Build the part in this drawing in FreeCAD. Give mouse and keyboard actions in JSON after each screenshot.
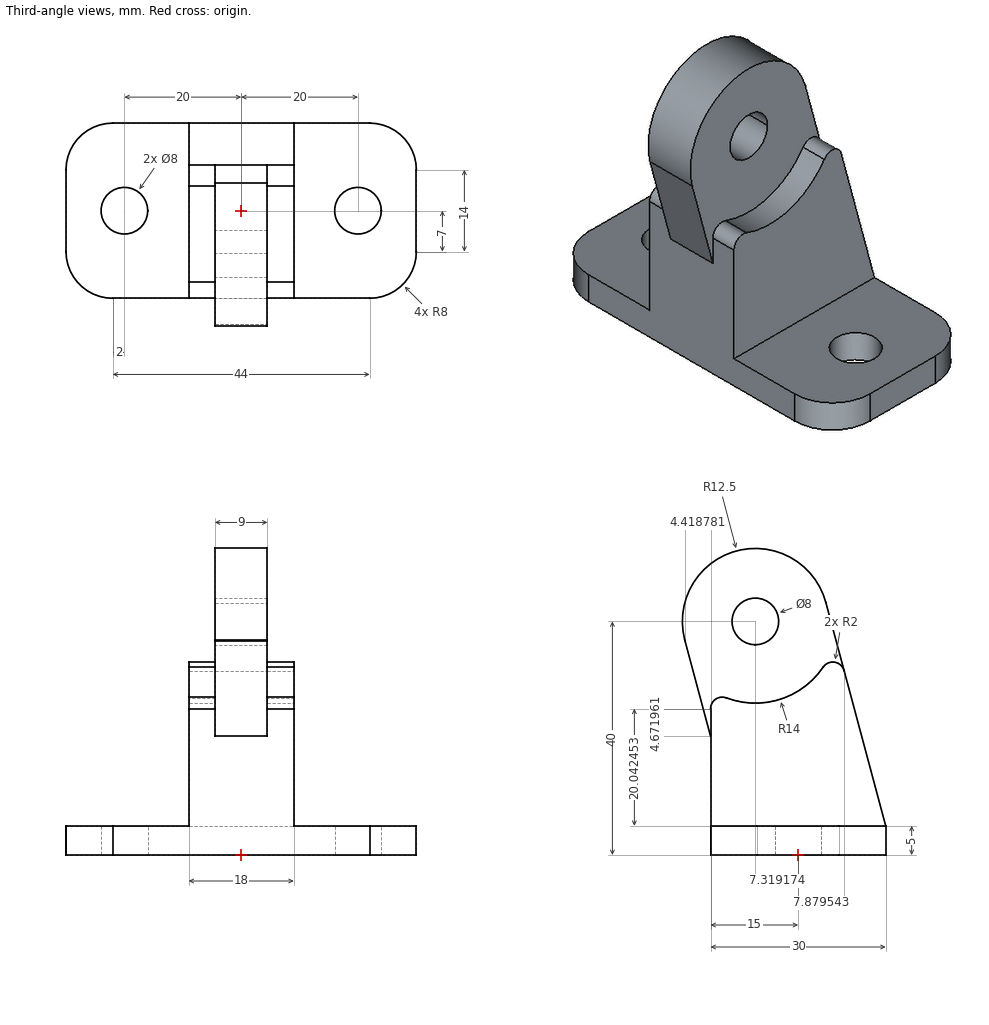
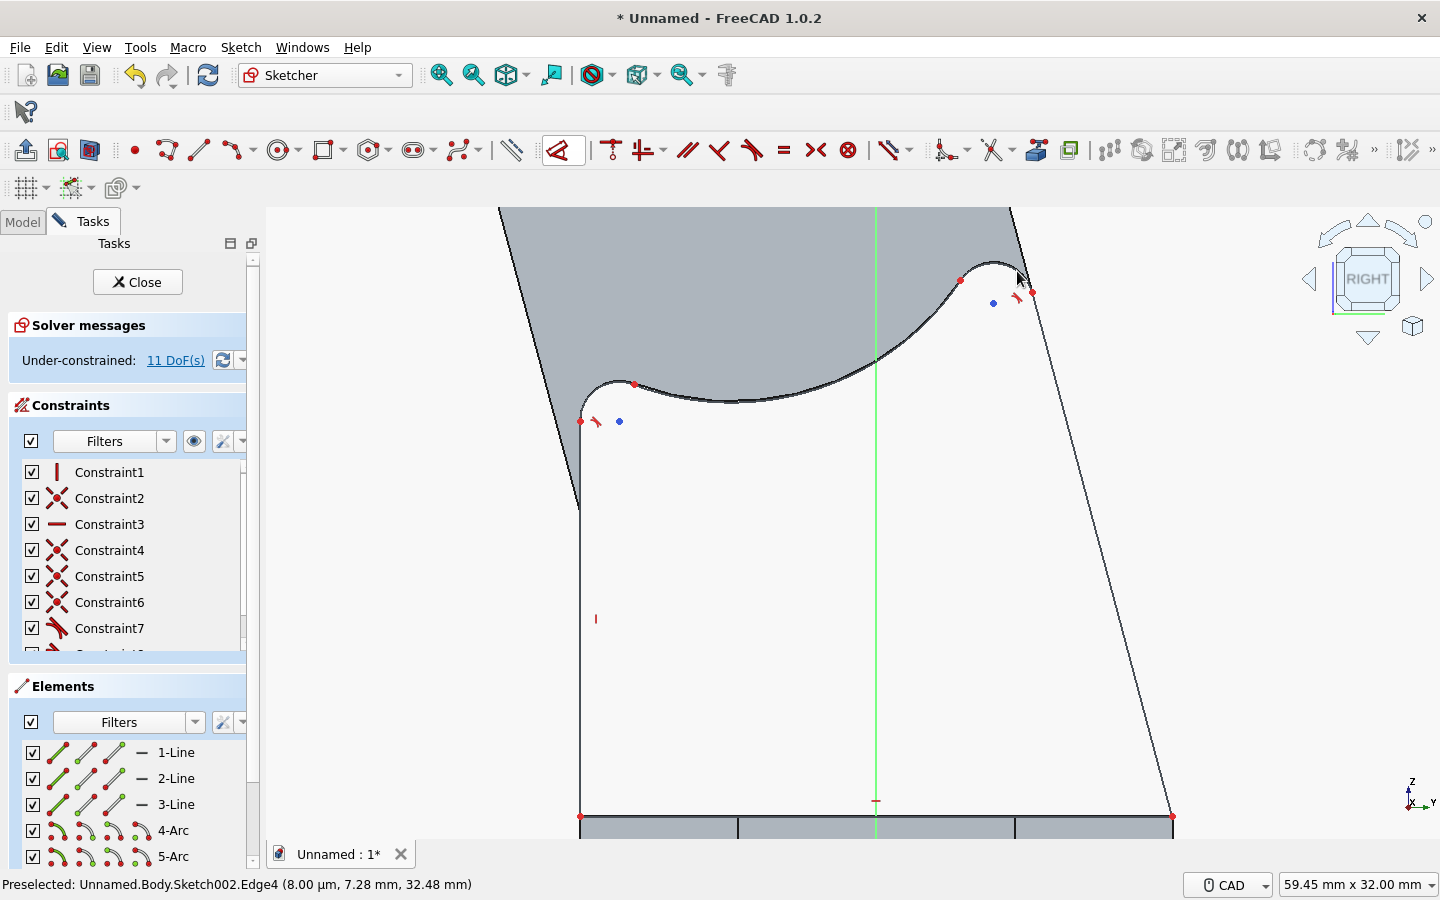
{"action": "left_click", "coordinate": [1017, 271]}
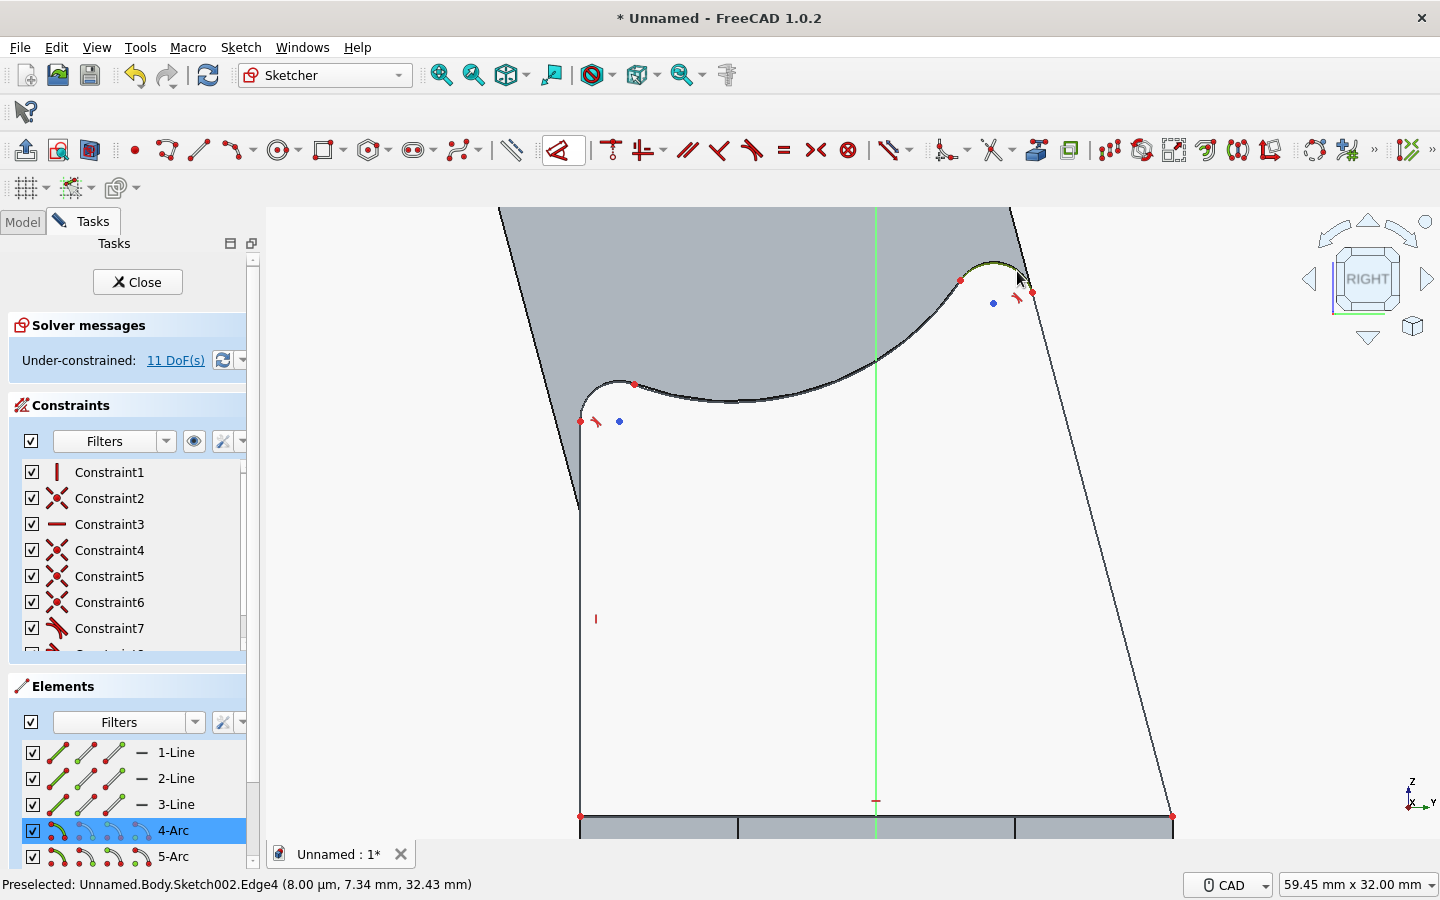
{"action": "left_click", "coordinate": [743, 402]}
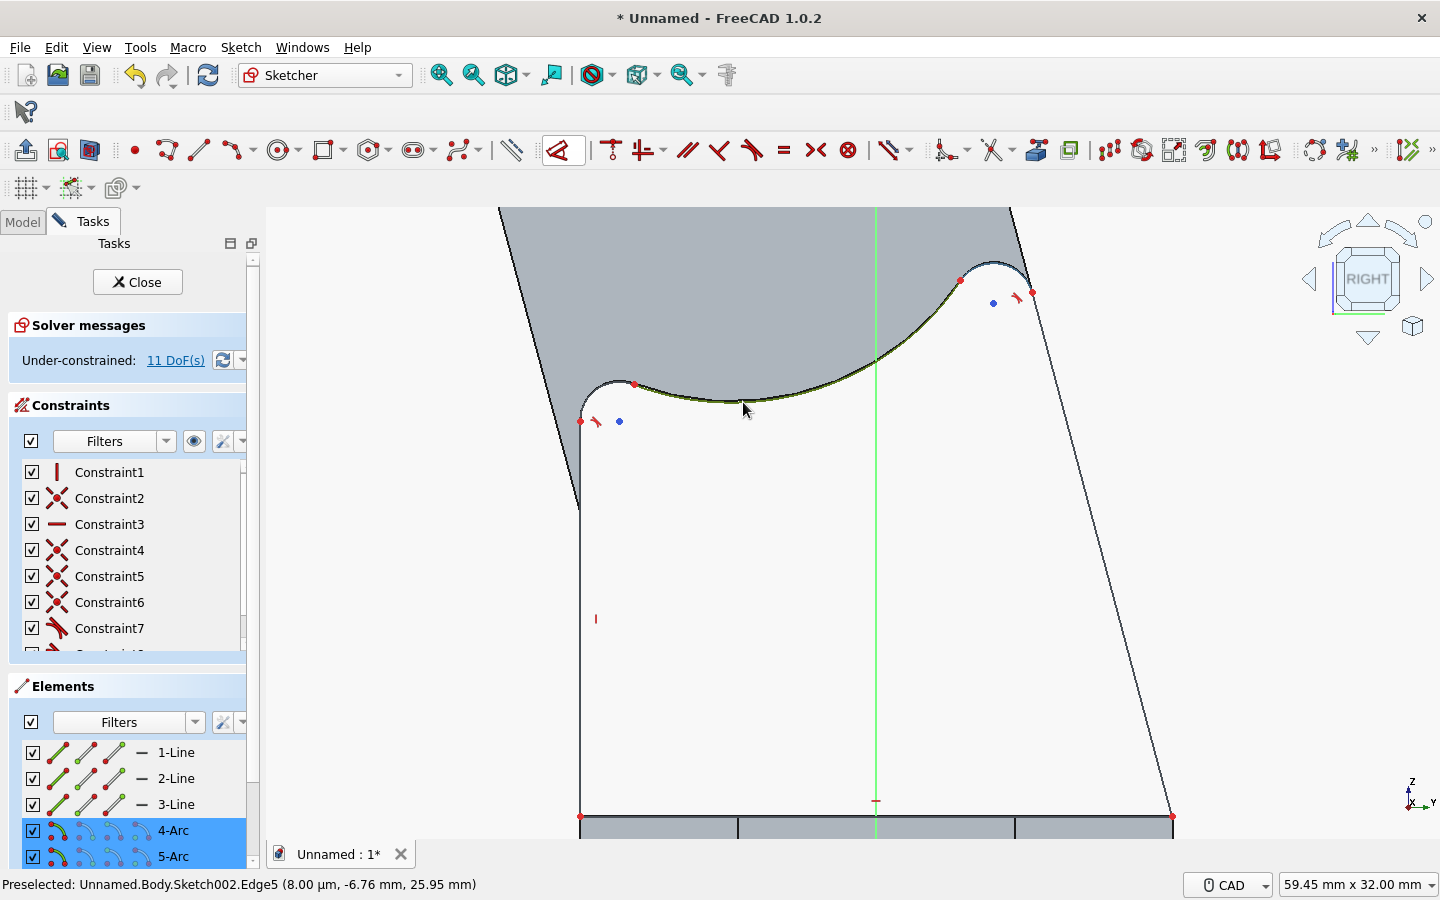
{"action": "key", "text": "t"}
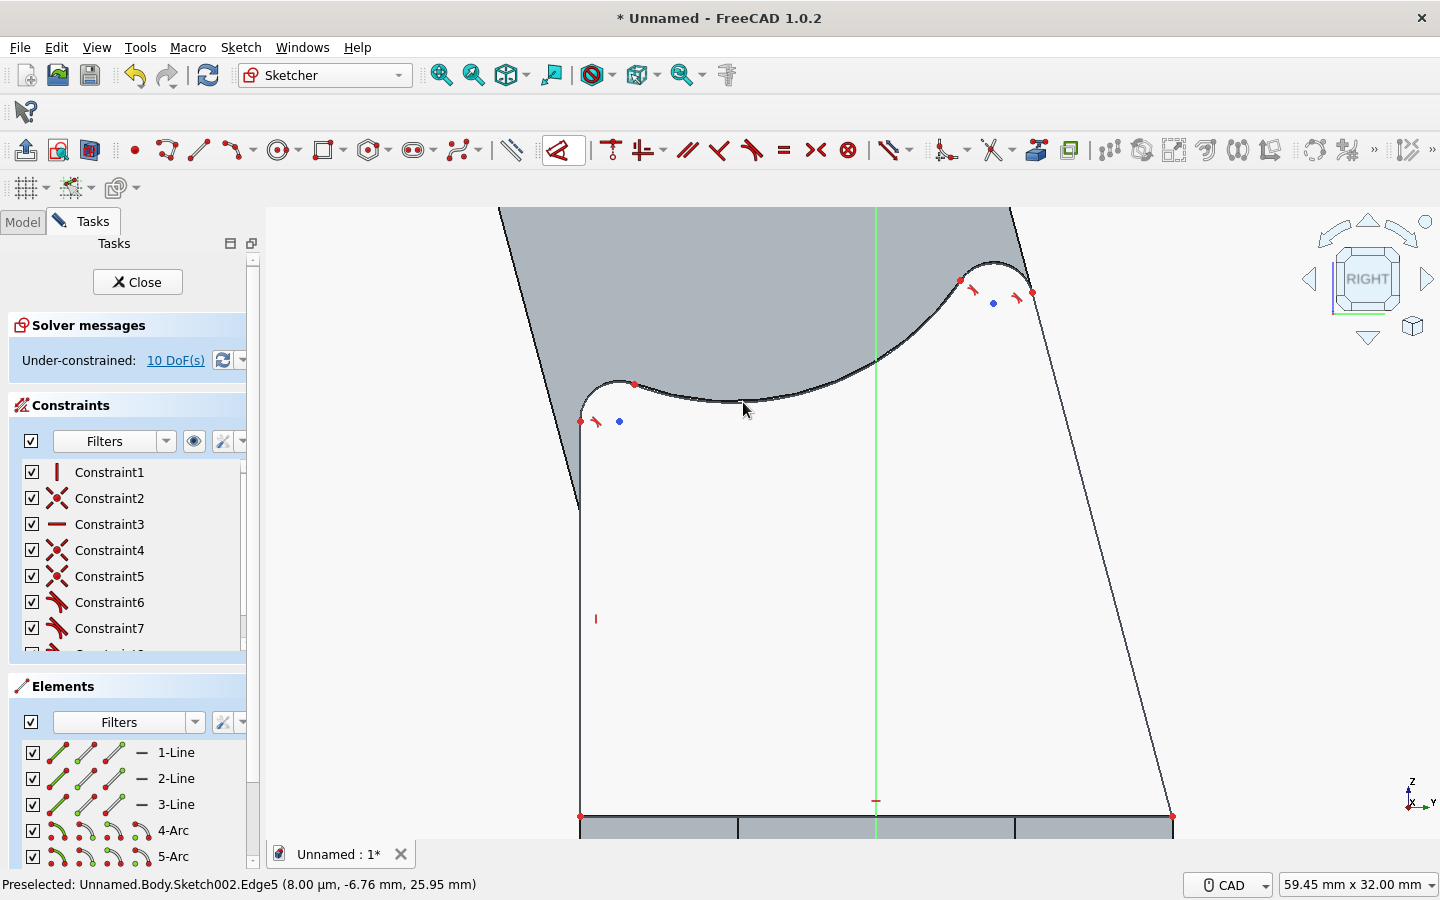
{"action": "left_click", "coordinate": [743, 402]}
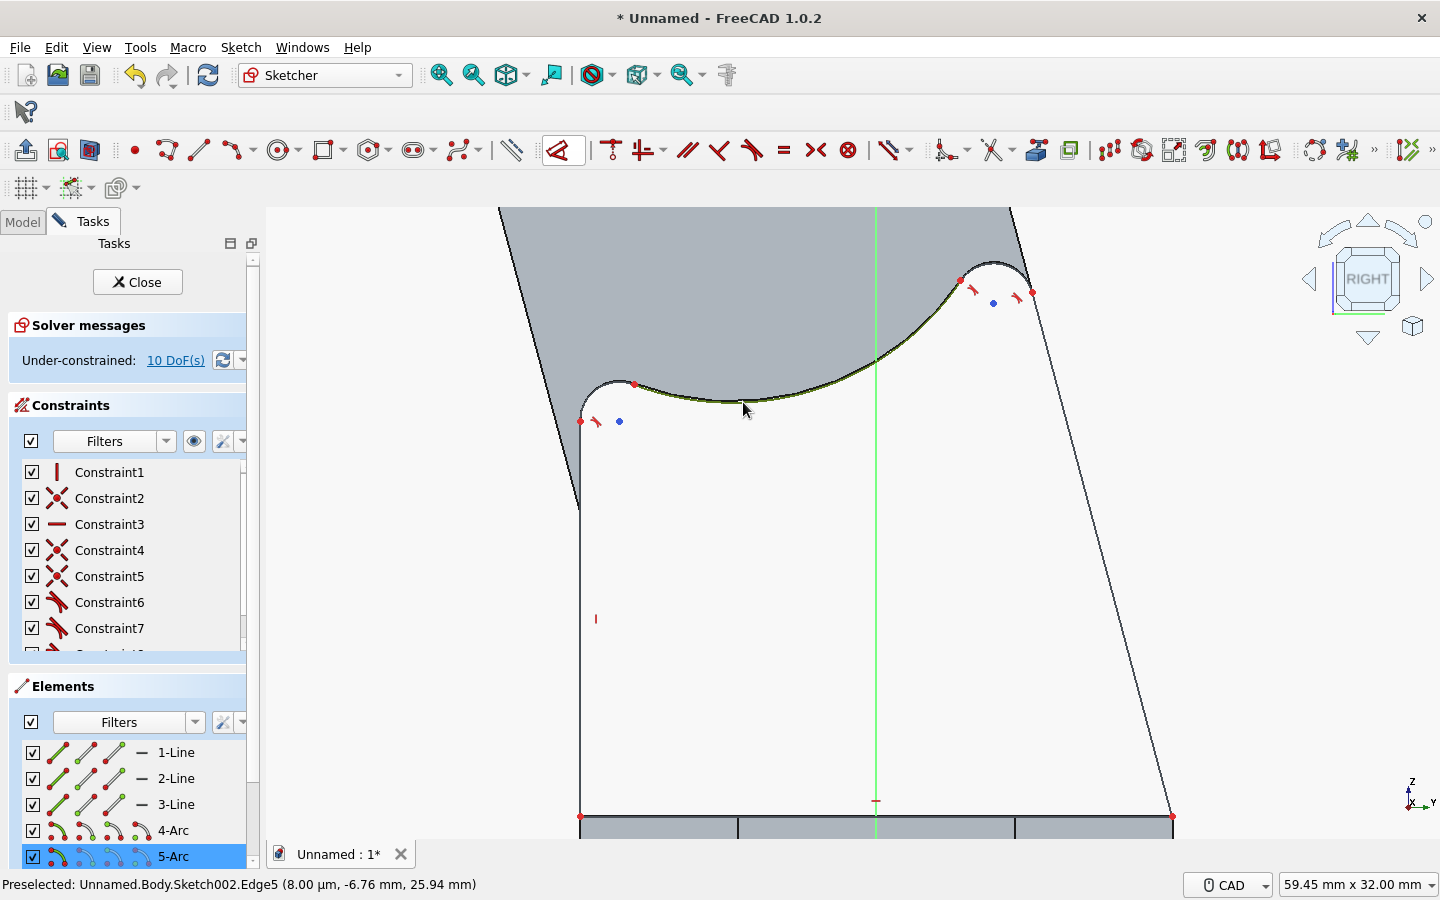
{"action": "left_click", "coordinate": [612, 383]}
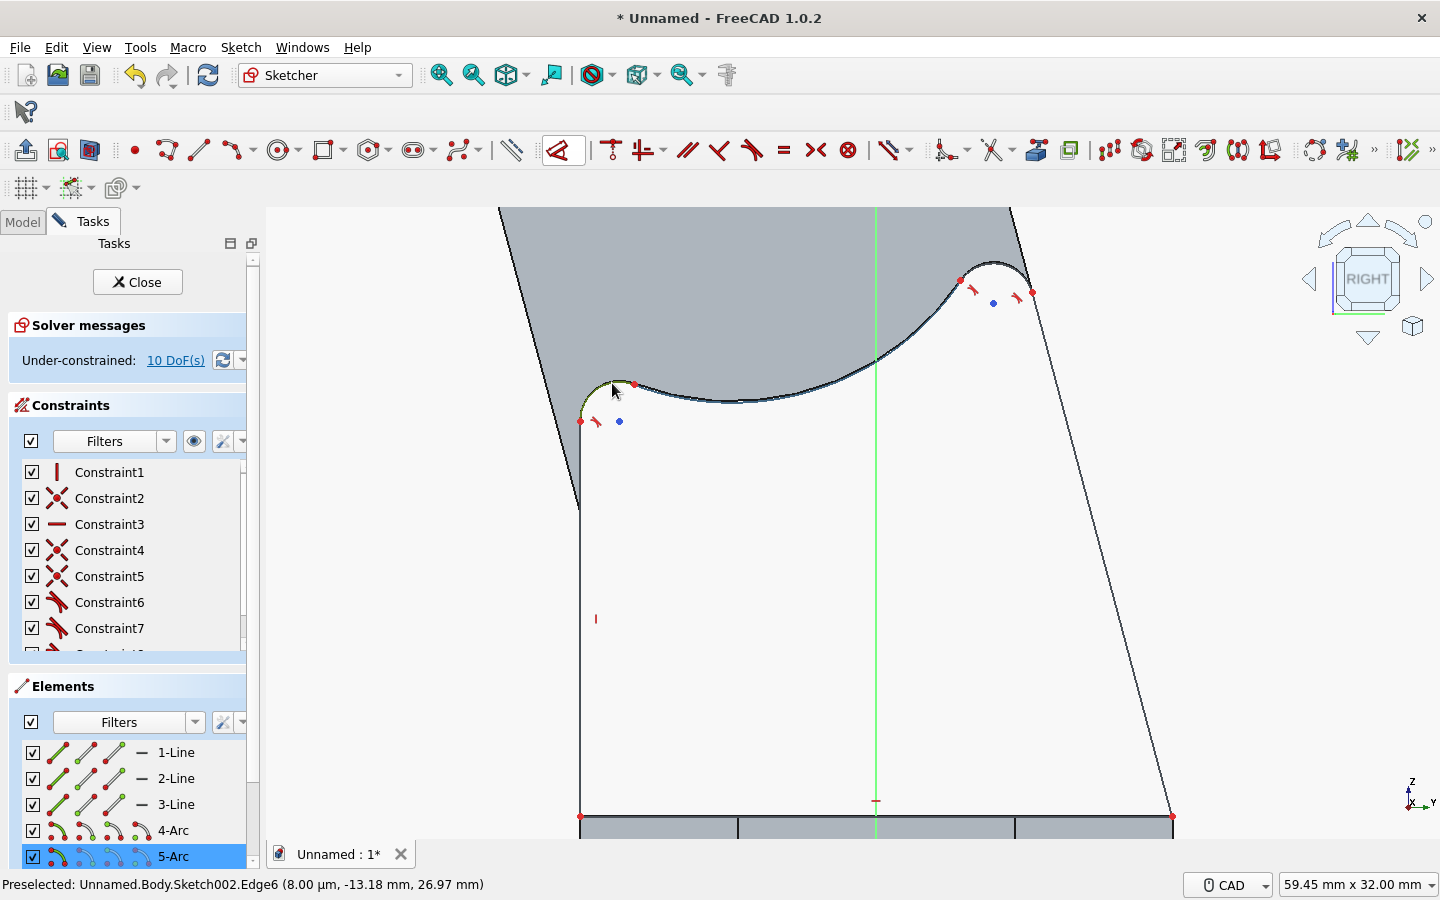
{"action": "key", "text": "t"}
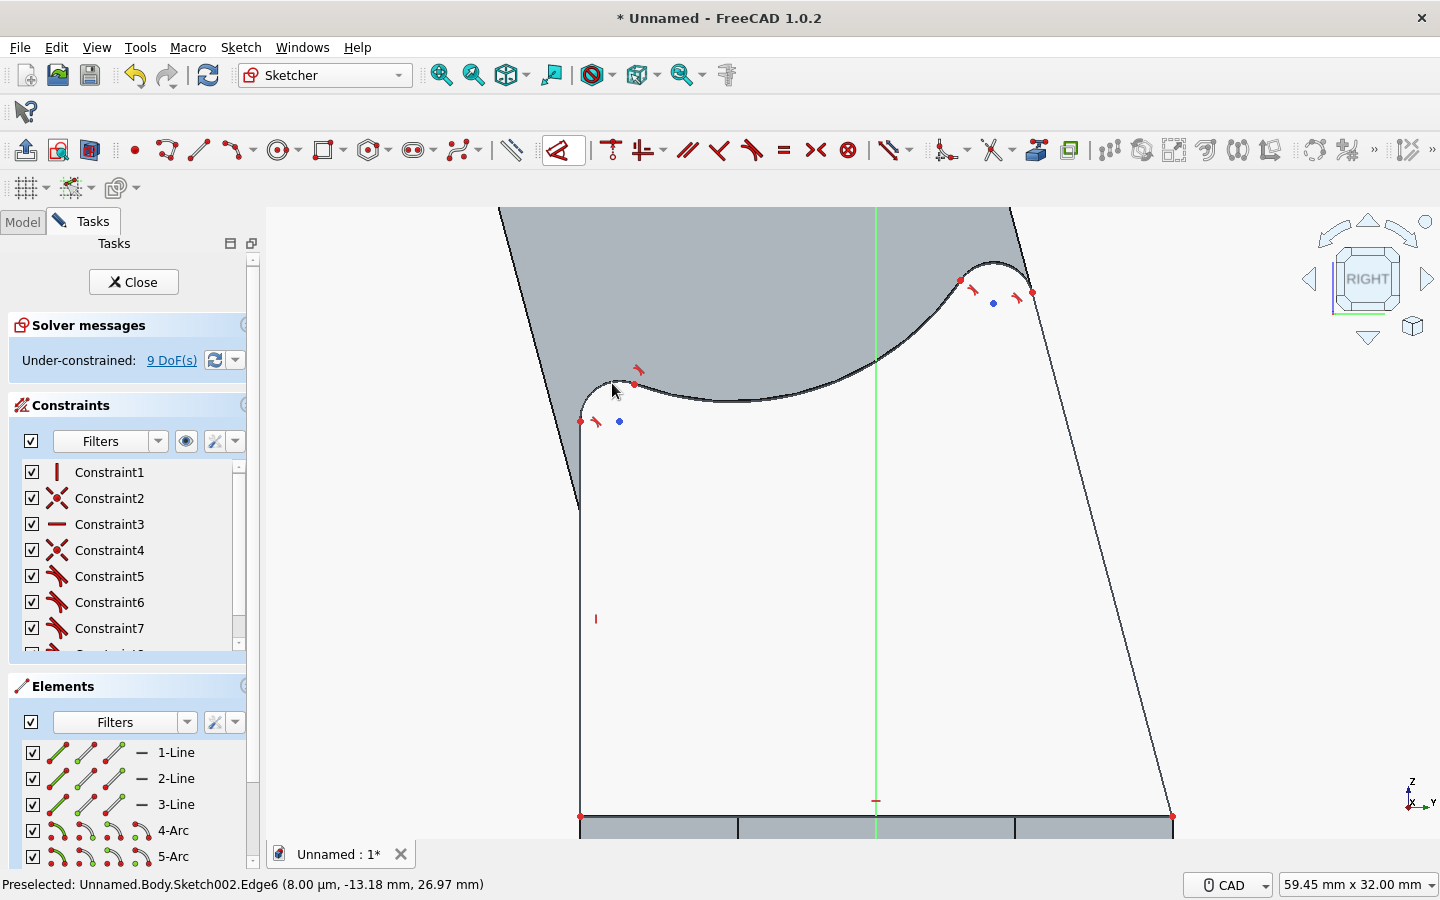
{"action": "left_click", "coordinate": [1017, 271]}